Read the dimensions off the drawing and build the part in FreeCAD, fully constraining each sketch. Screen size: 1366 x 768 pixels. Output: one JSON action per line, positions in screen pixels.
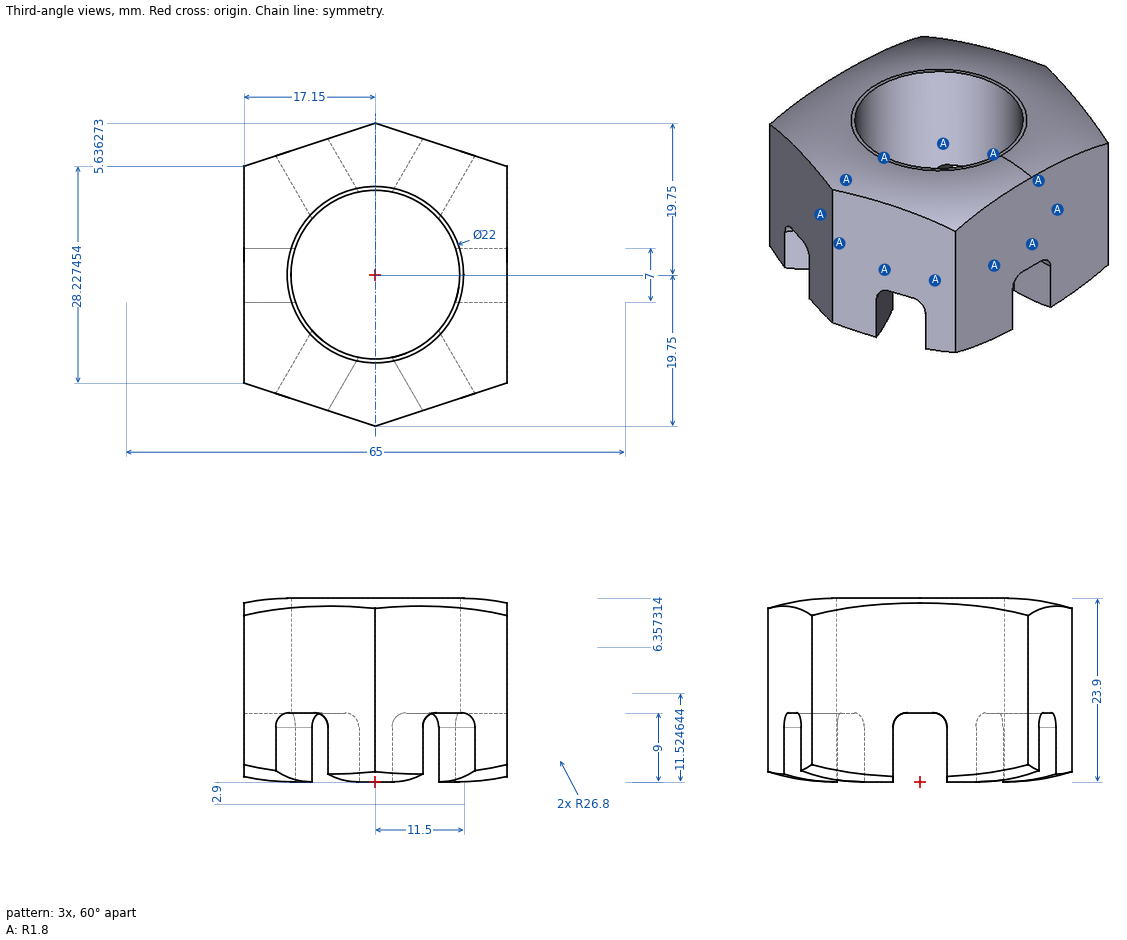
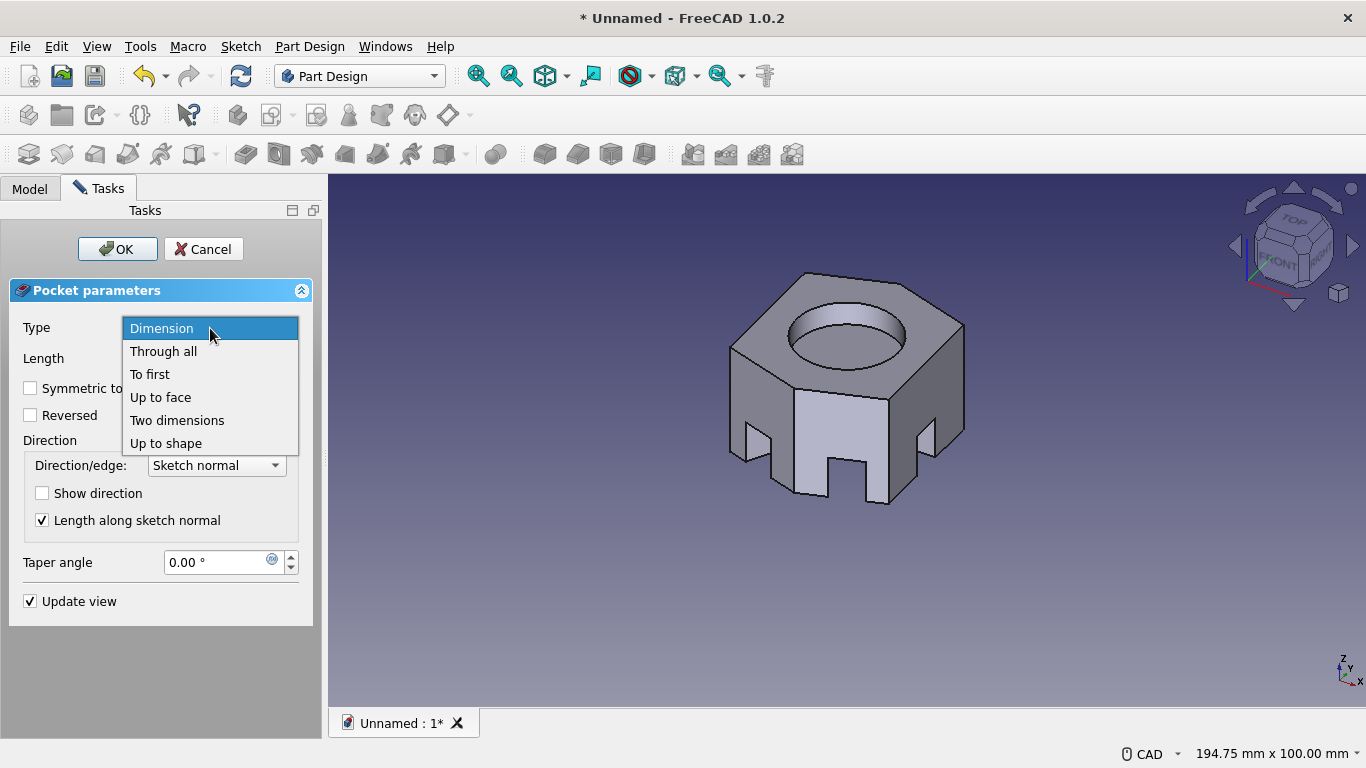
{"action": "left_click", "coordinate": [208, 352]}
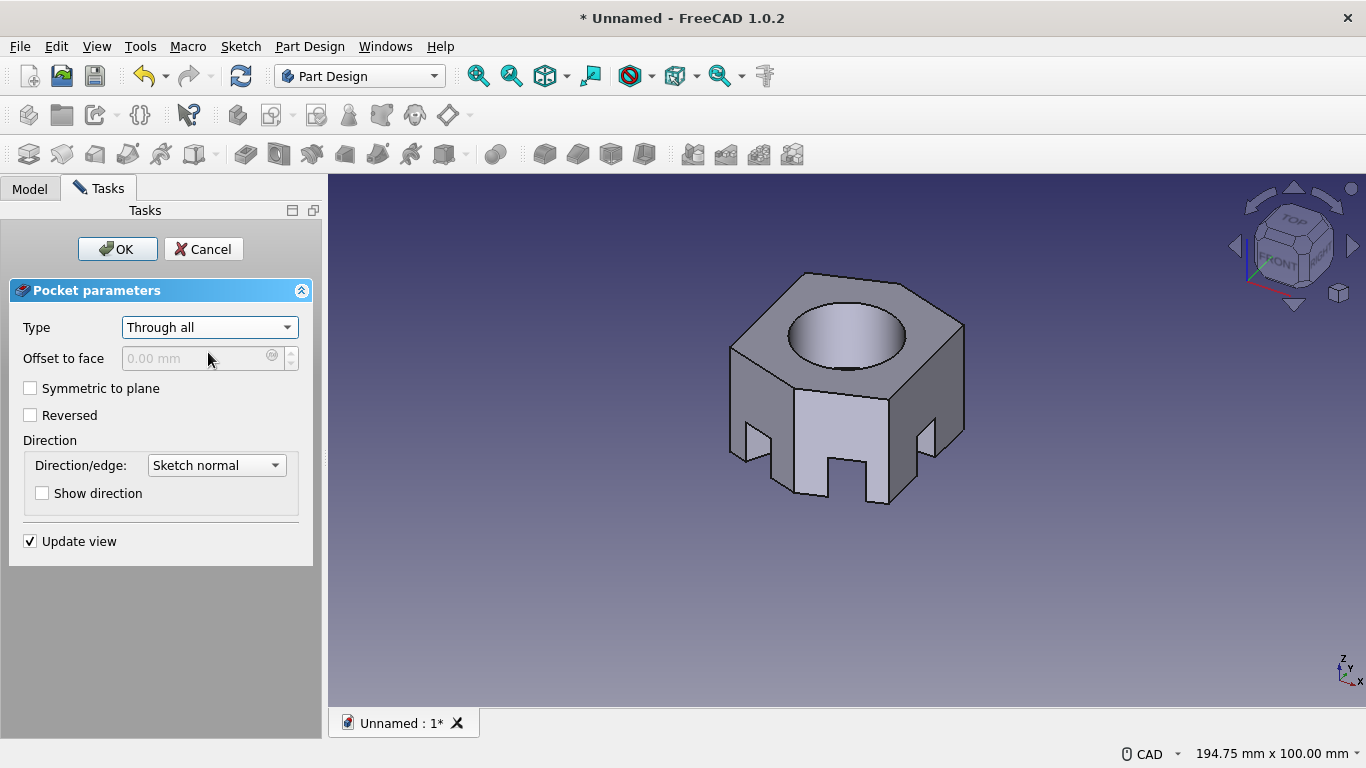
{"action": "left_click", "coordinate": [118, 249]}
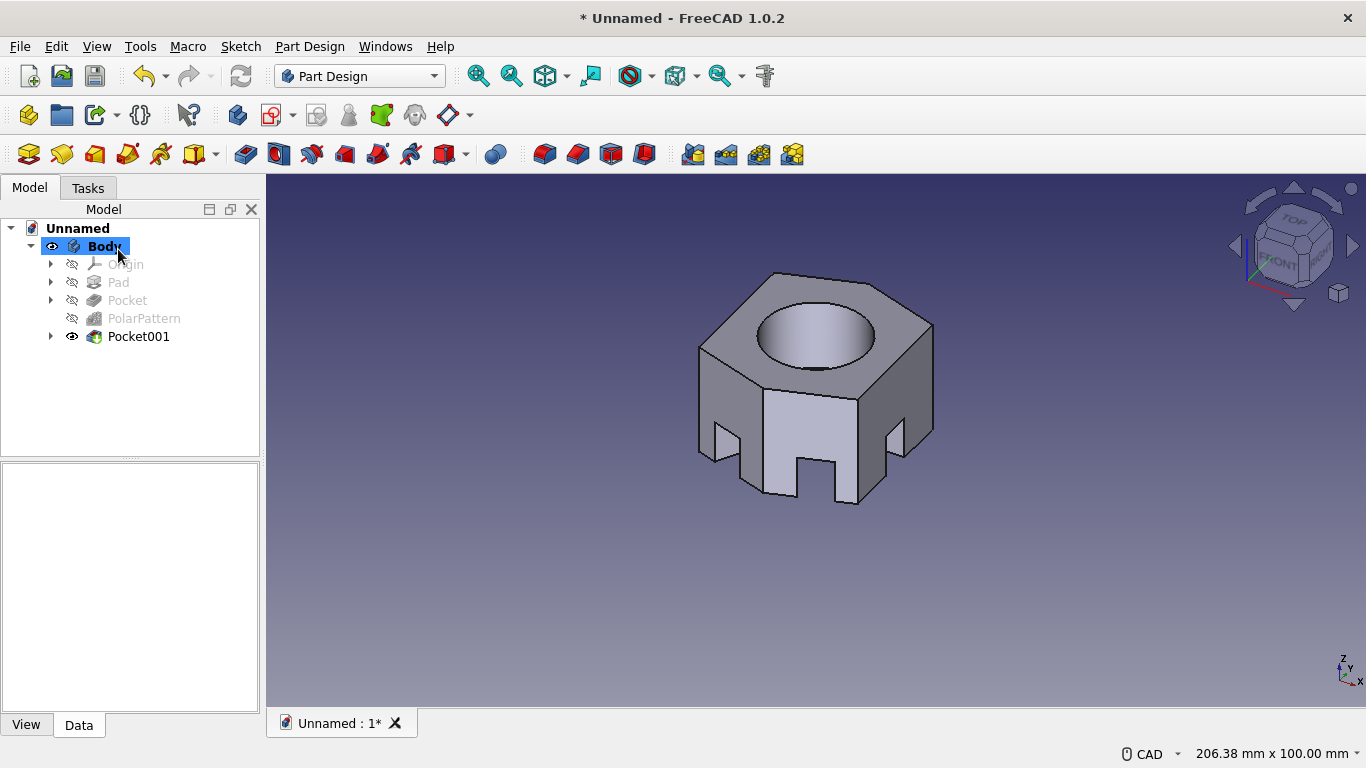
{"action": "key", "text": "0"}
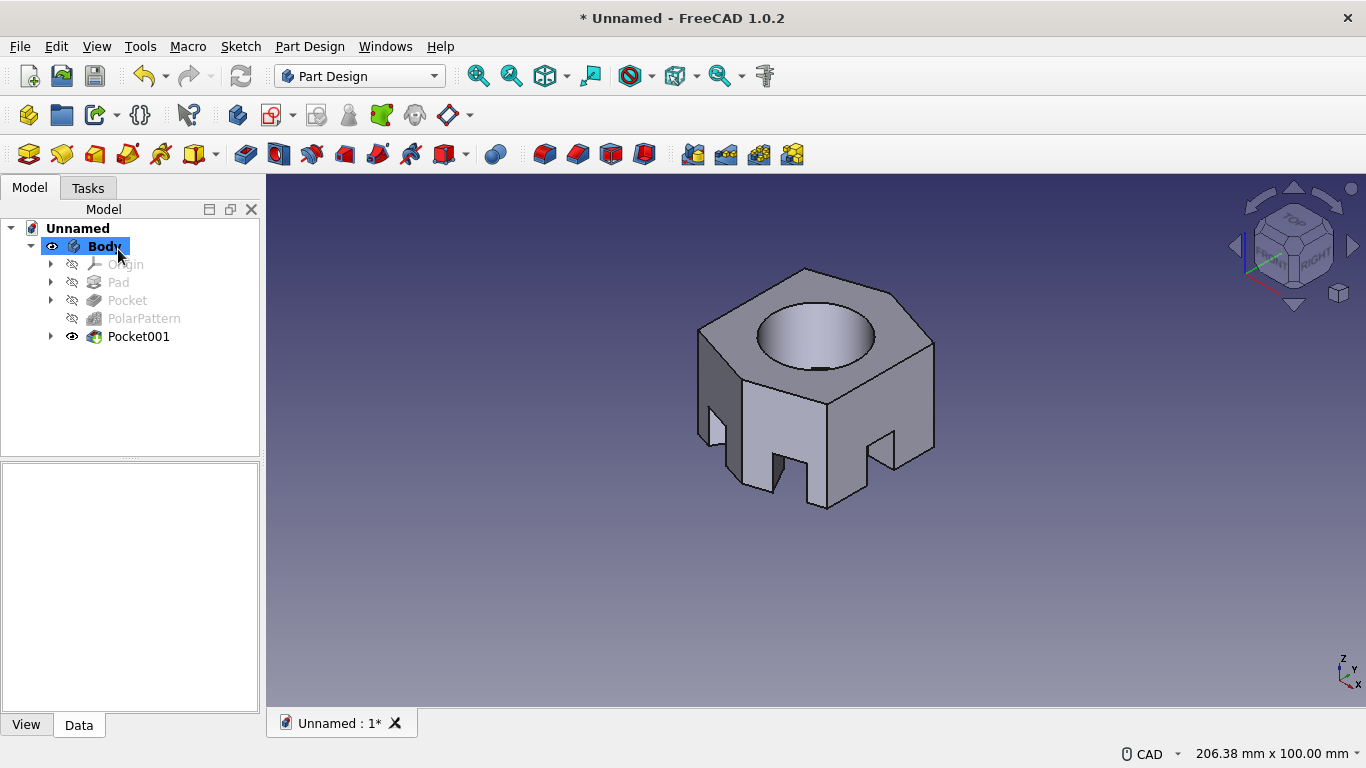
{"action": "key", "text": "2"}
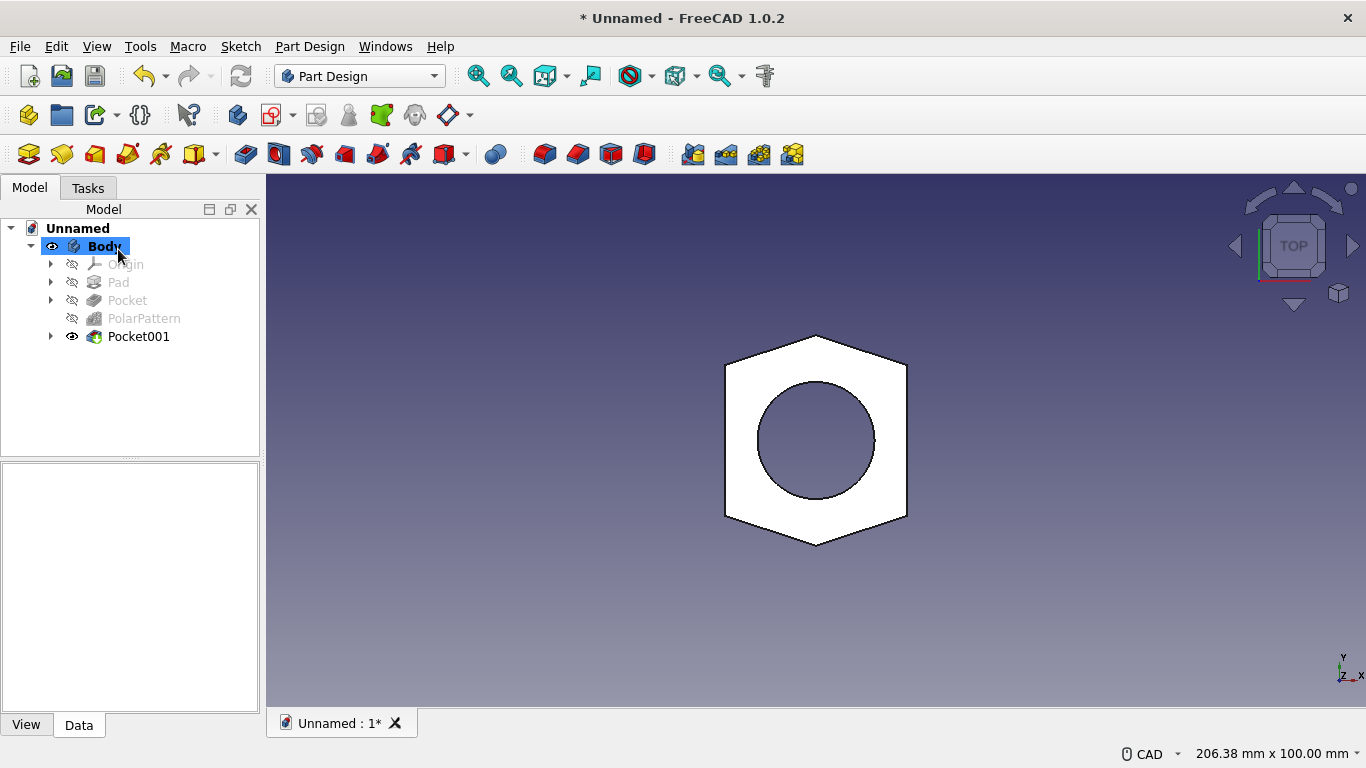
{"action": "left_click", "coordinate": [479, 76]}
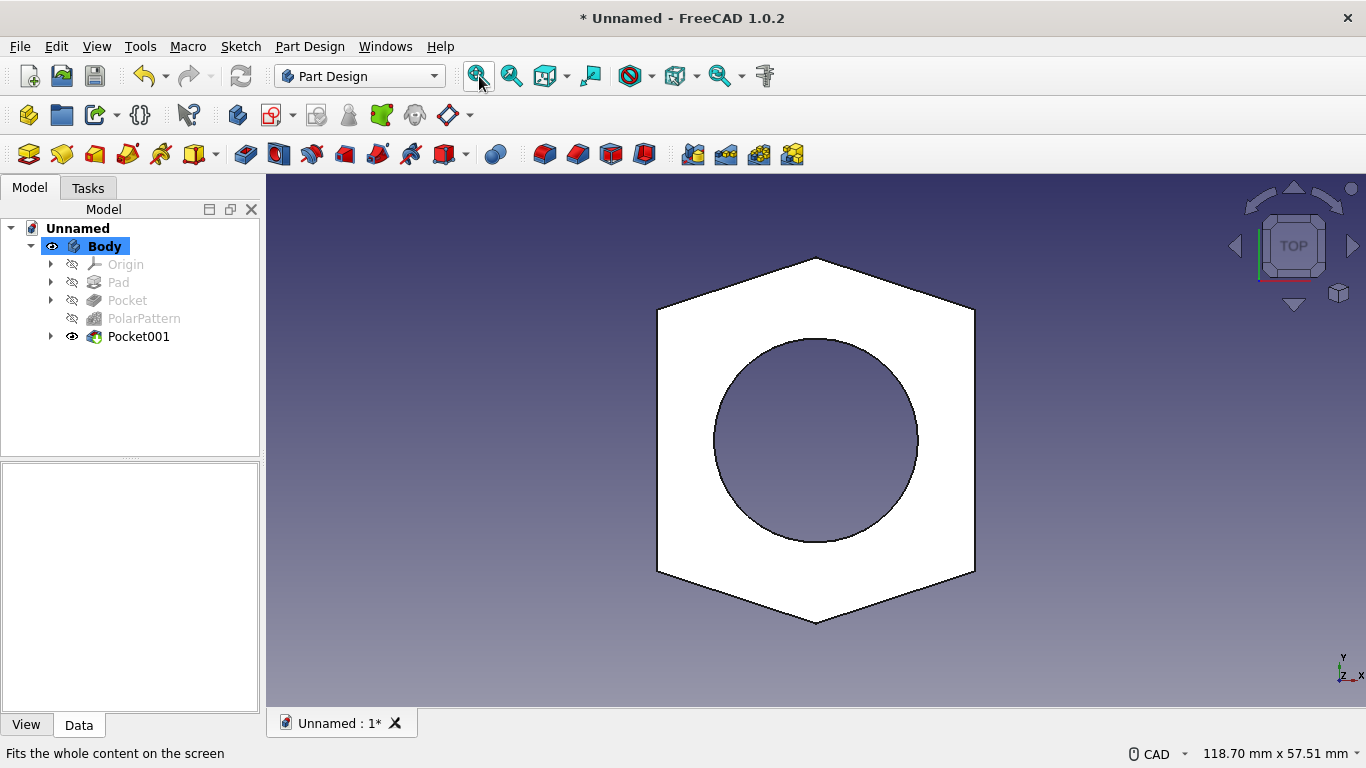
{"action": "key", "text": "1"}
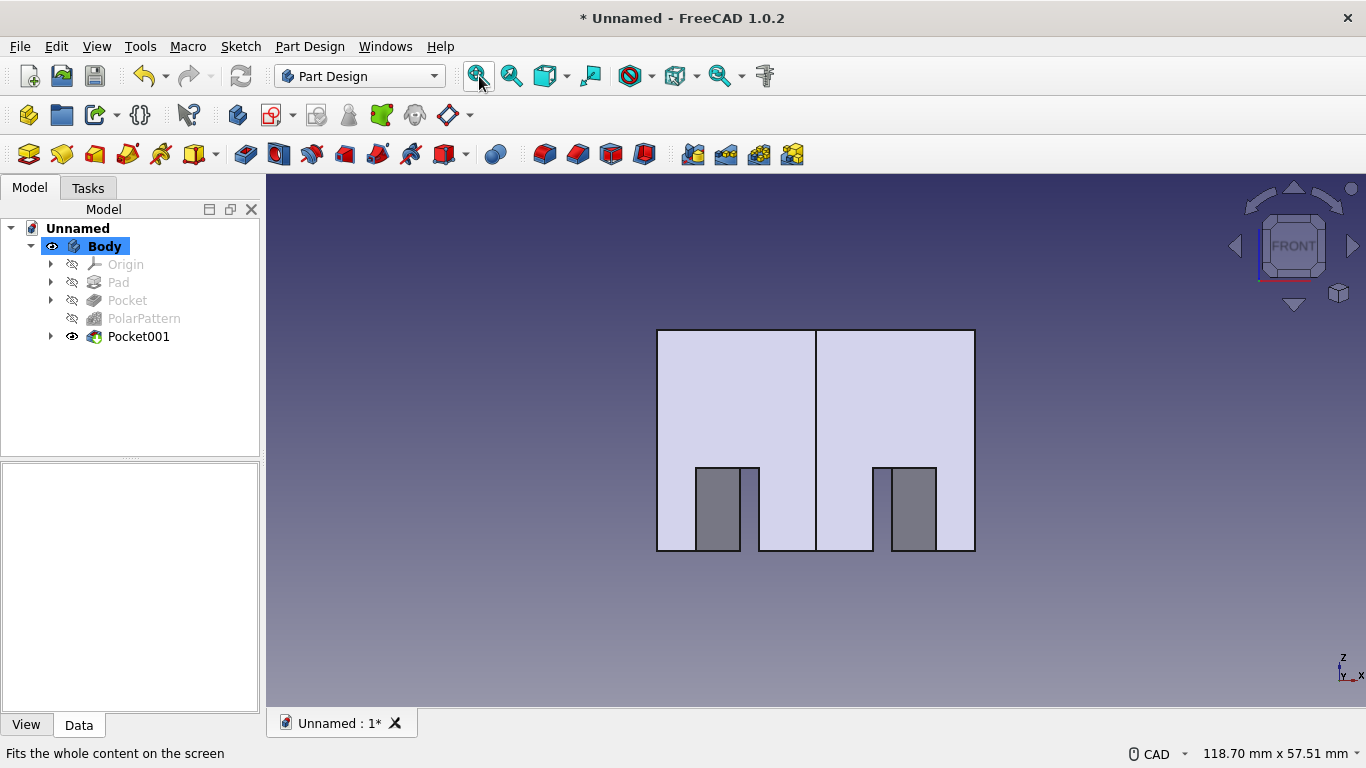
{"action": "left_click", "coordinate": [479, 76]}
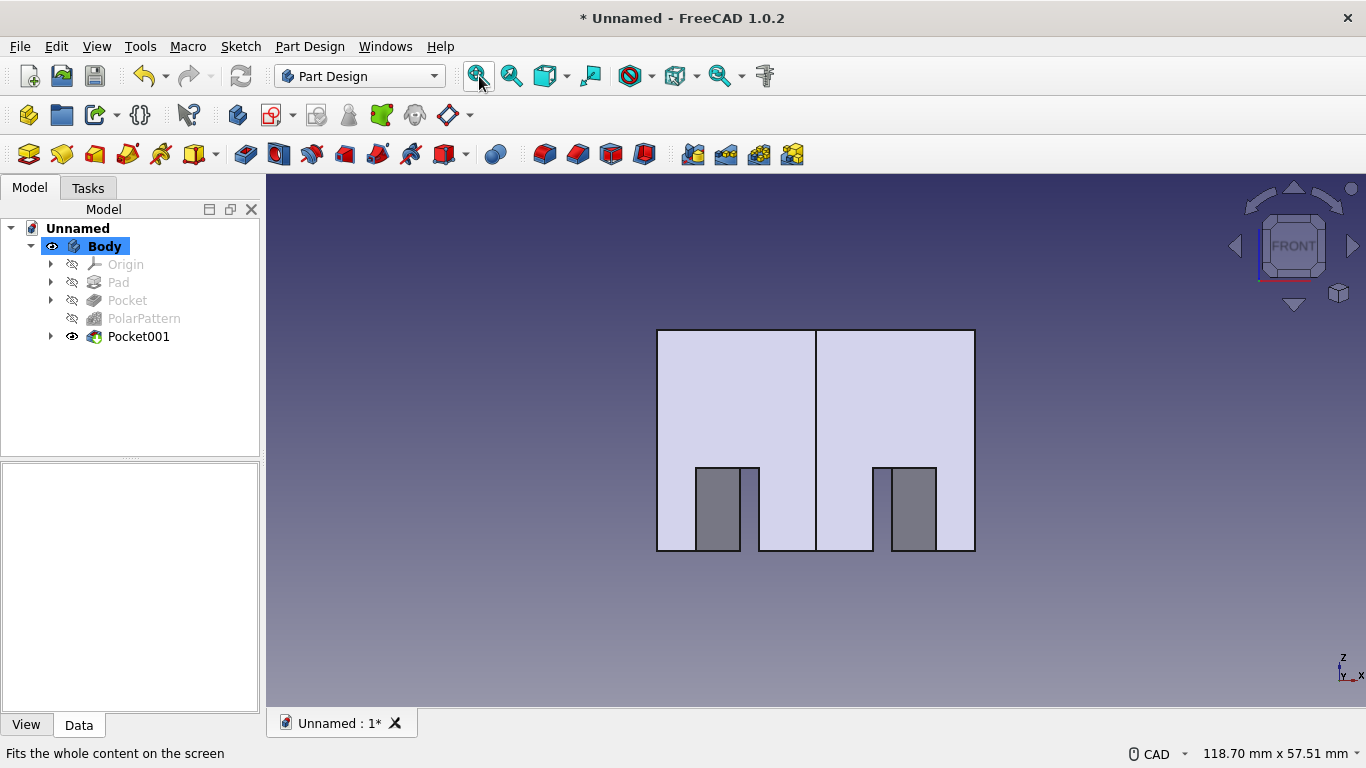
{"action": "key", "text": "3"}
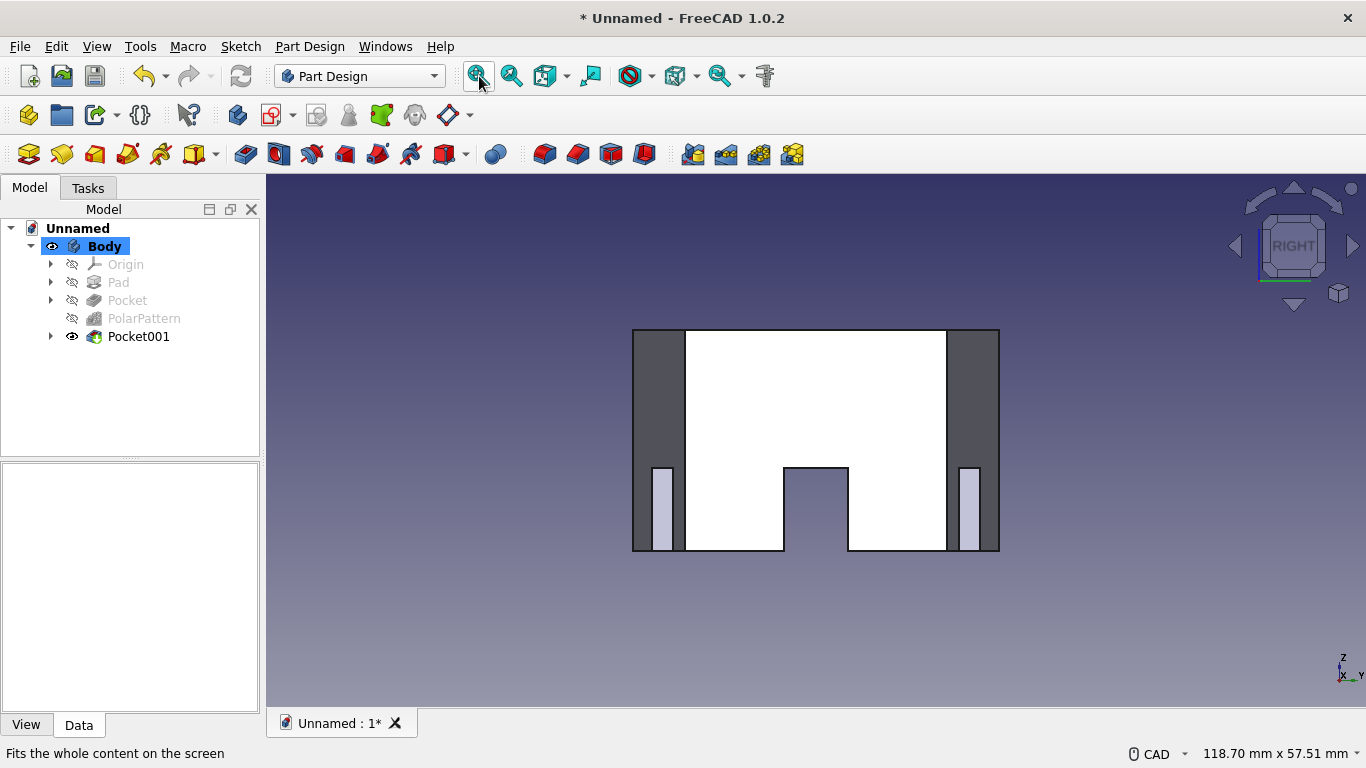
{"action": "left_click", "coordinate": [479, 76]}